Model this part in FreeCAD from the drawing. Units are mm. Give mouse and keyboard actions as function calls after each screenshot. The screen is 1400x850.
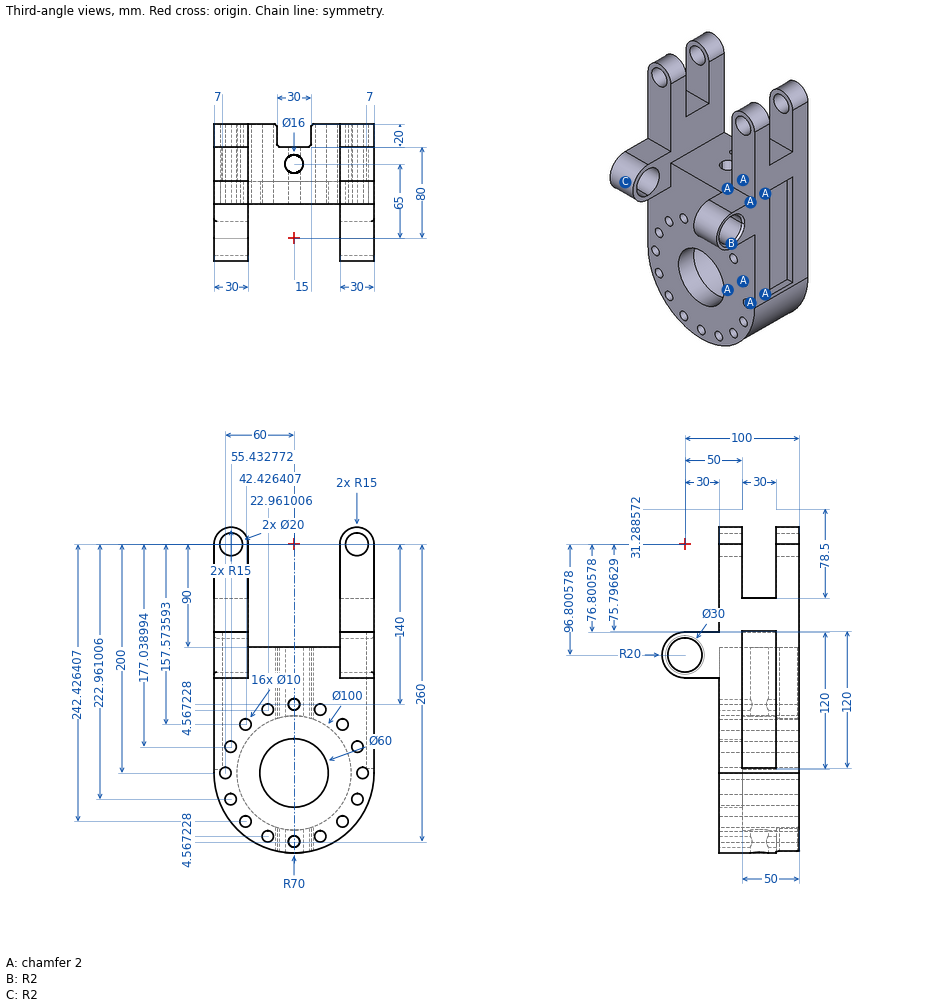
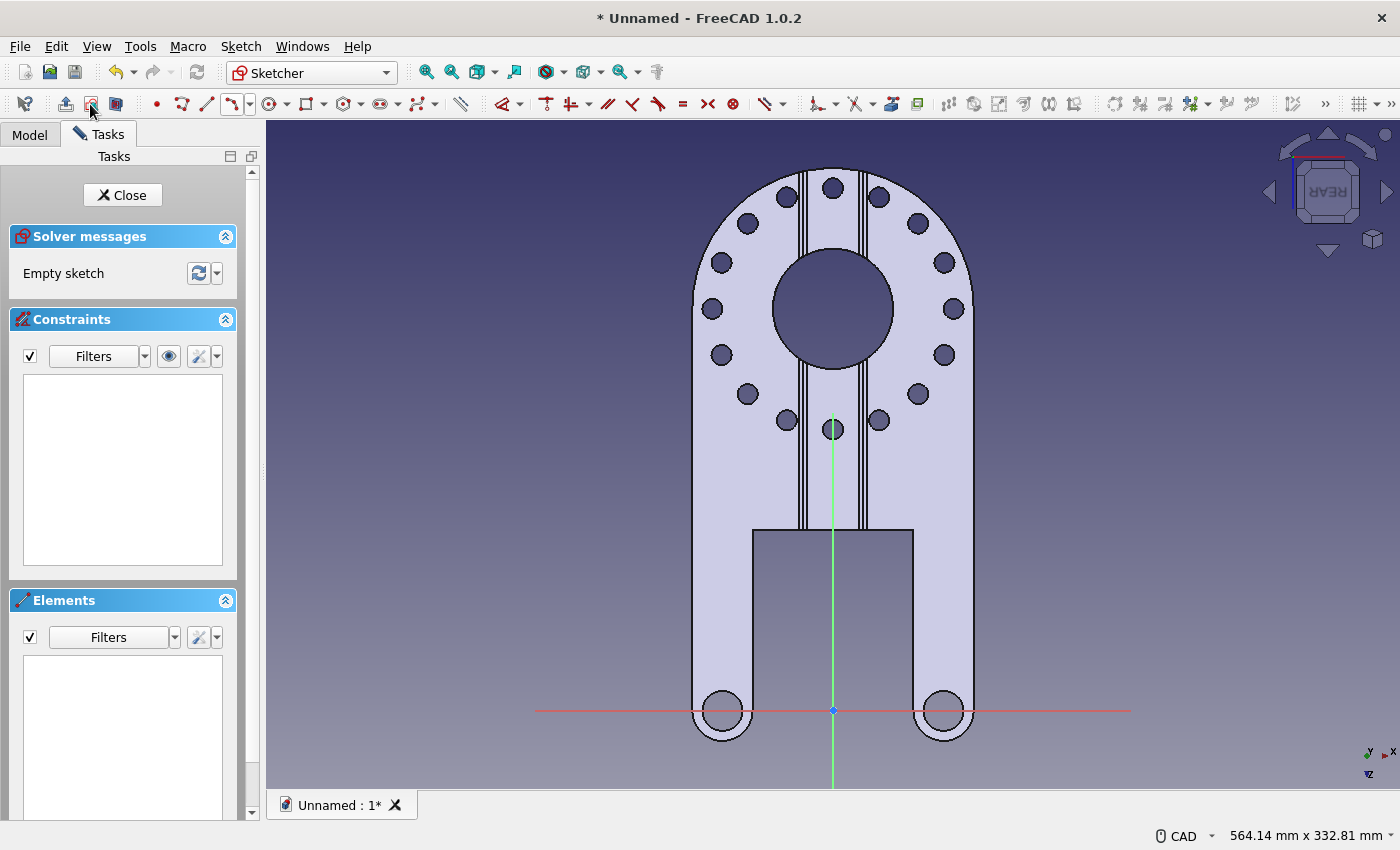
scroll(889, 190, up, 4)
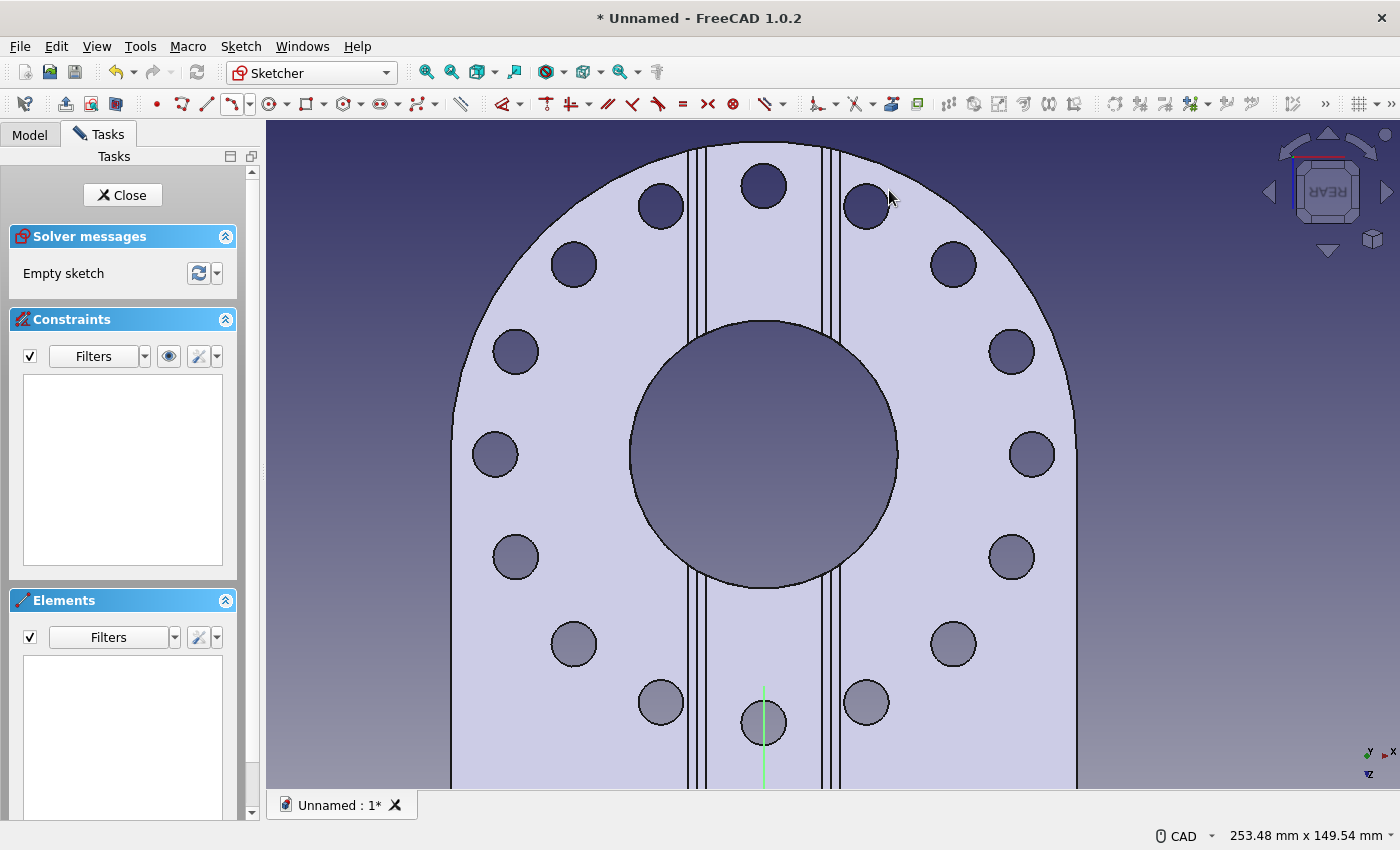
click(268, 104)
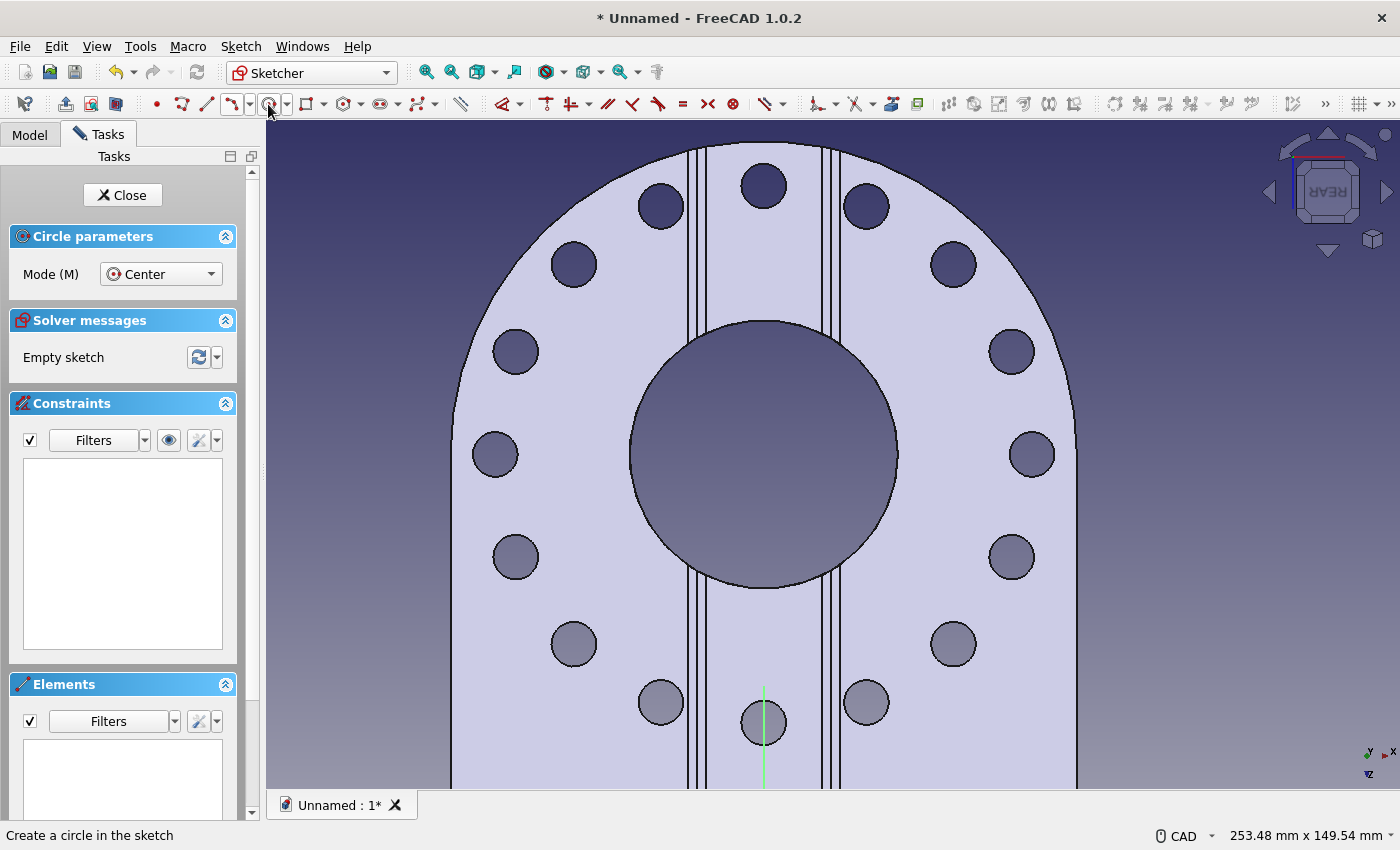
click(764, 454)
click(922, 296)
key(Escape)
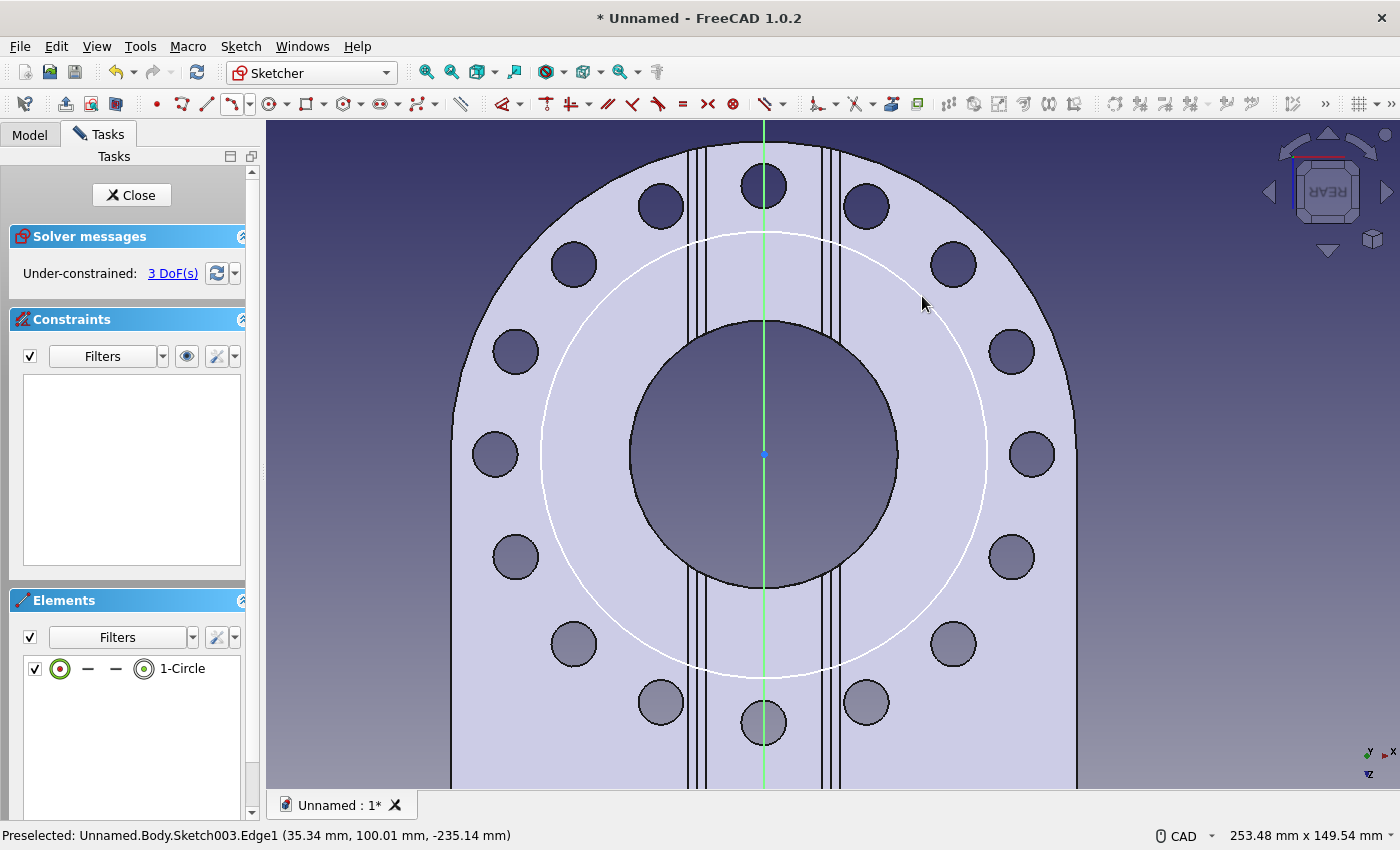
click(764, 455)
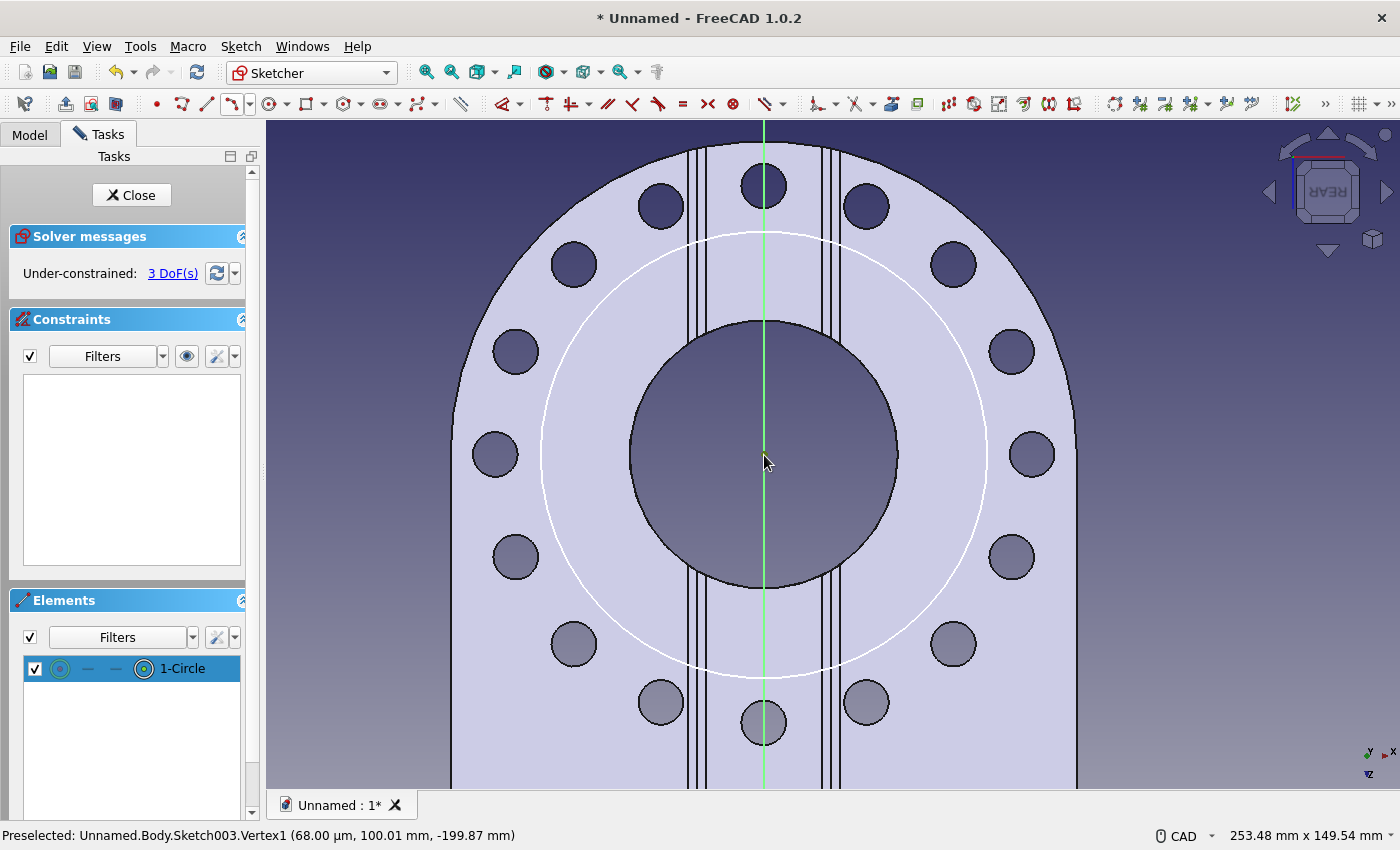
click(764, 717)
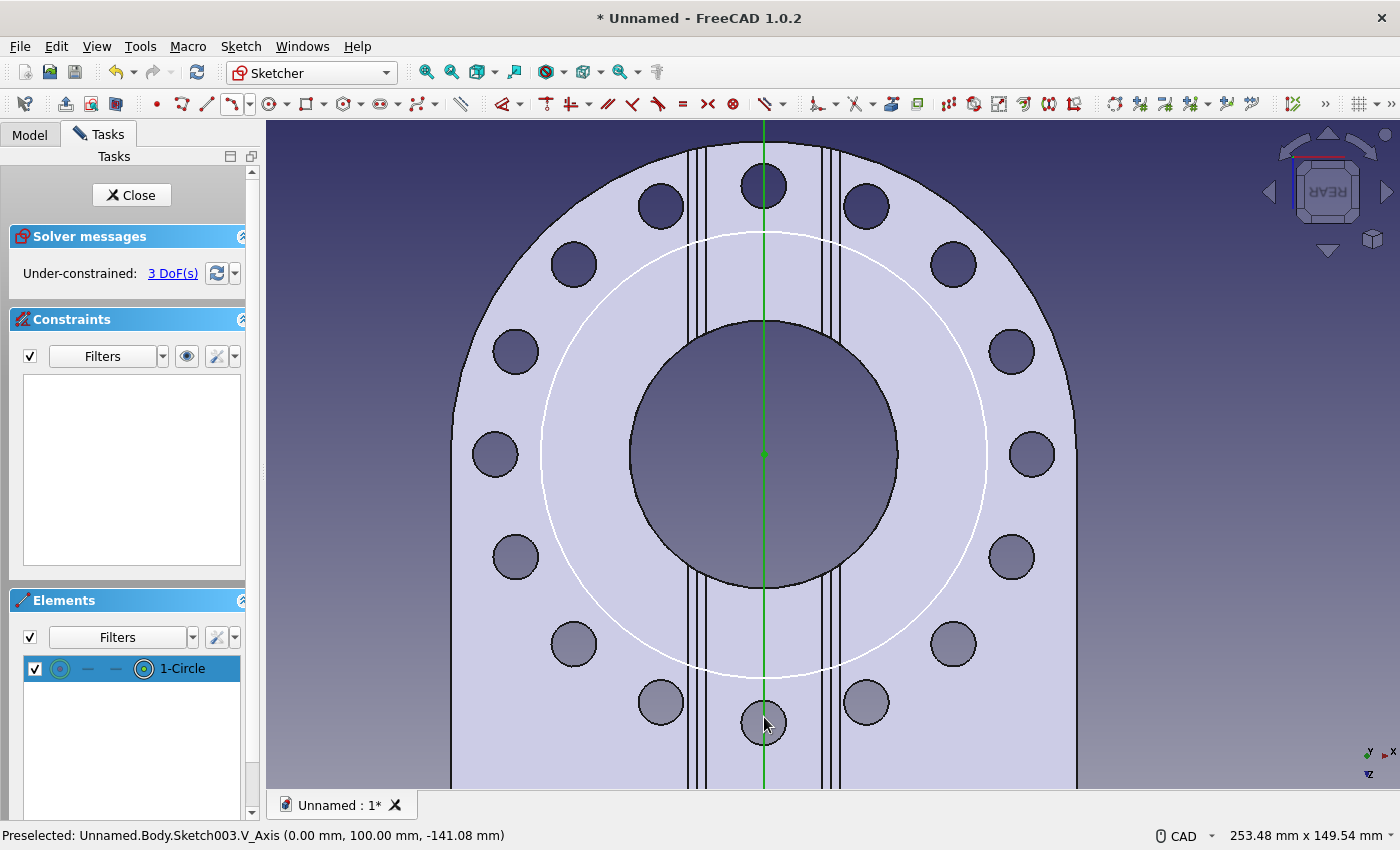
click(546, 104)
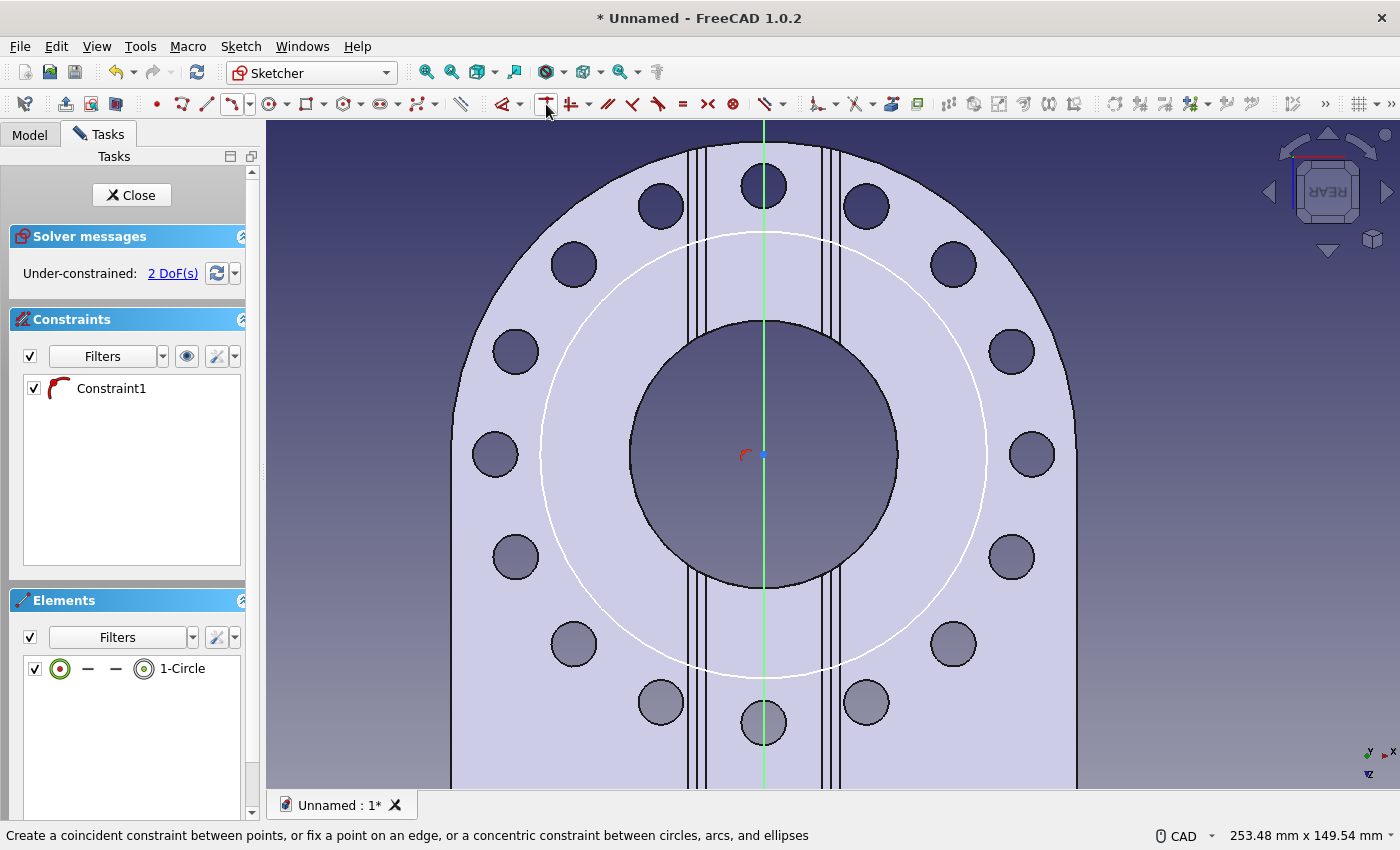
key(d)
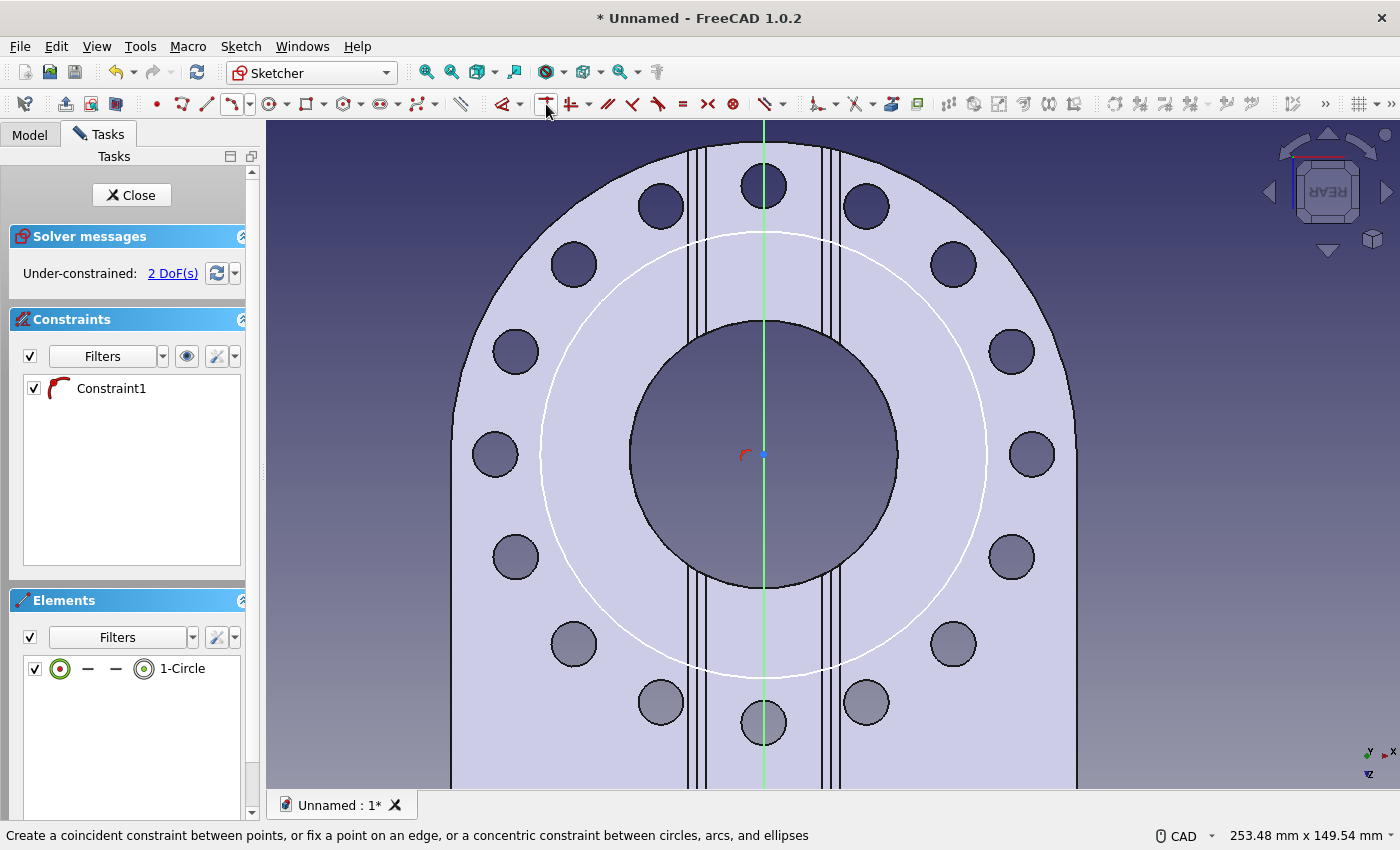
click(921, 297)
click(944, 274)